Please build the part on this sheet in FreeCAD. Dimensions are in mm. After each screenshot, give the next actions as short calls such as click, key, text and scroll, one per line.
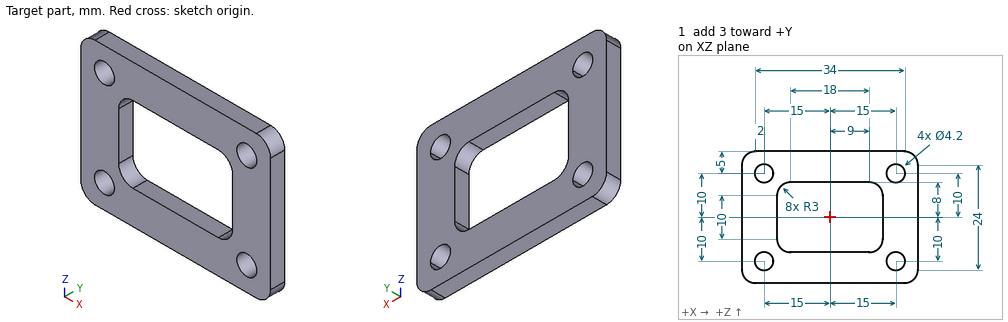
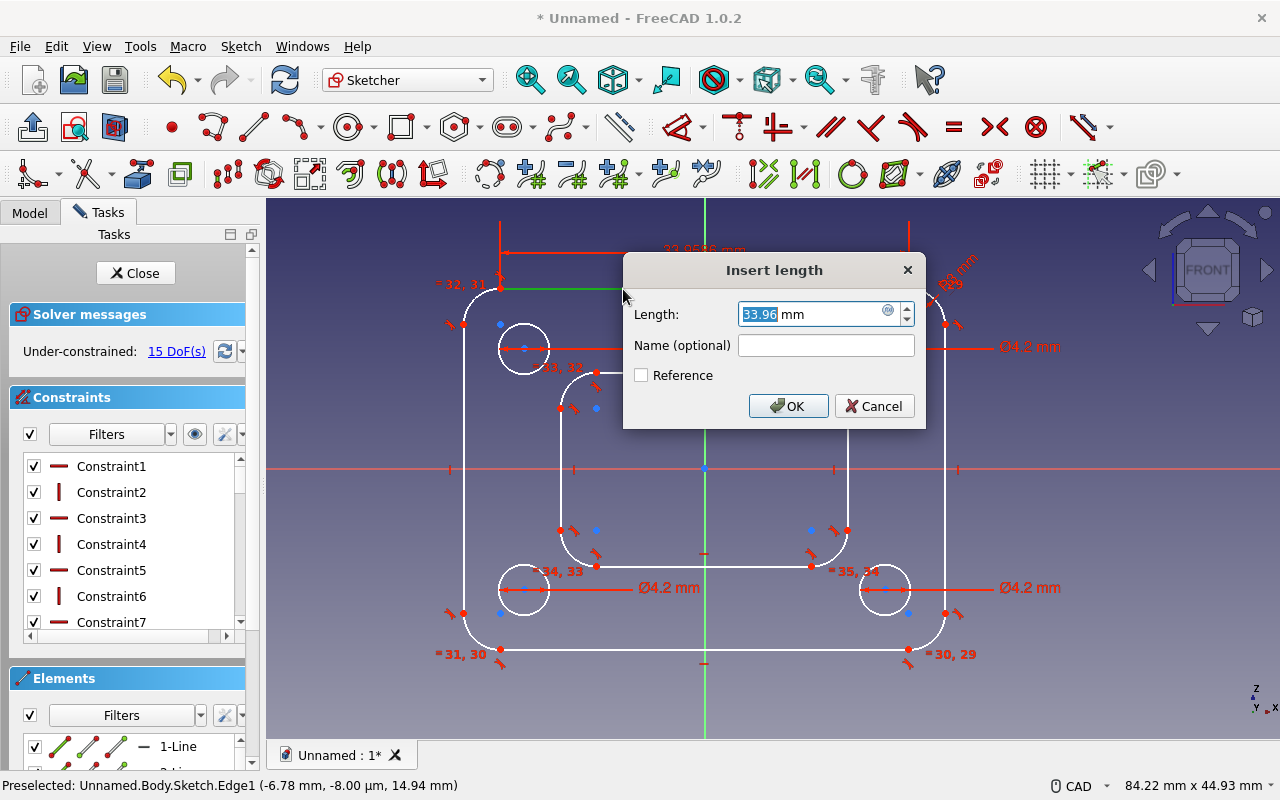
text(34)
key(Return)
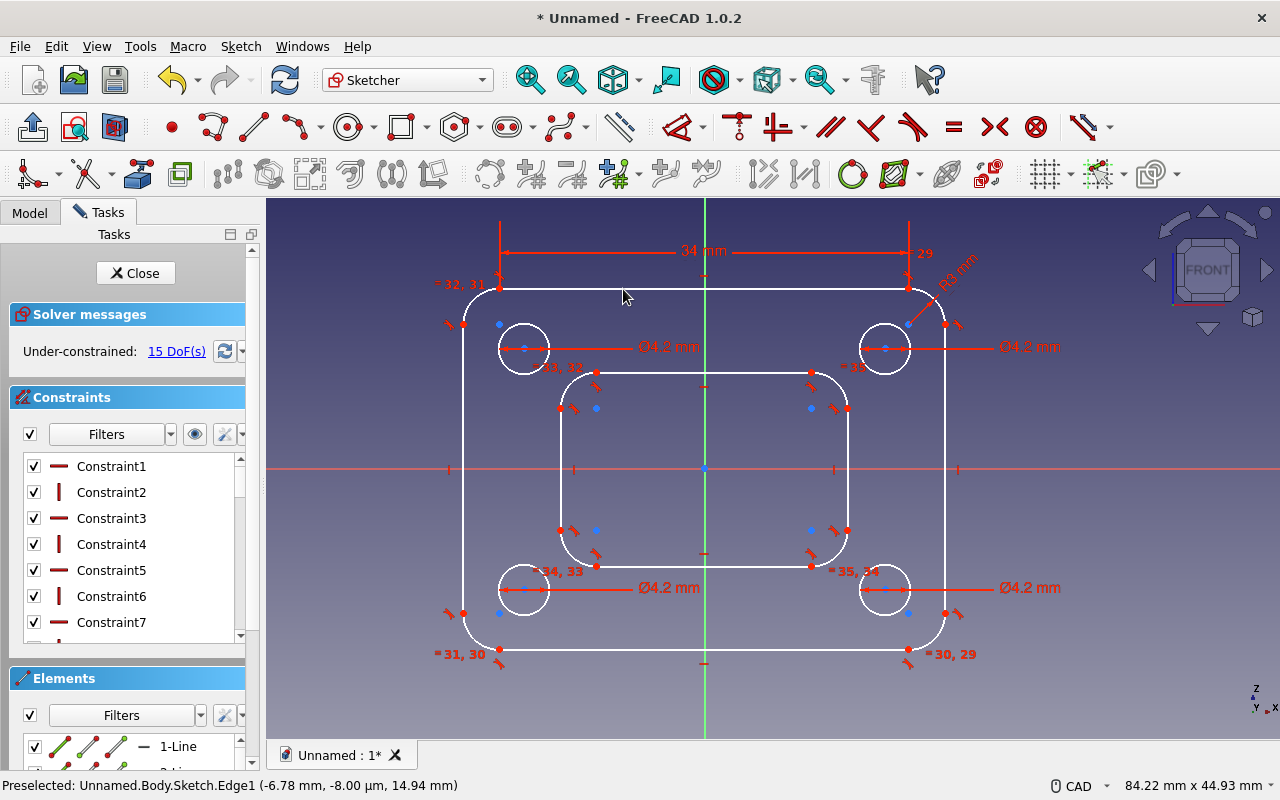
click(945, 412)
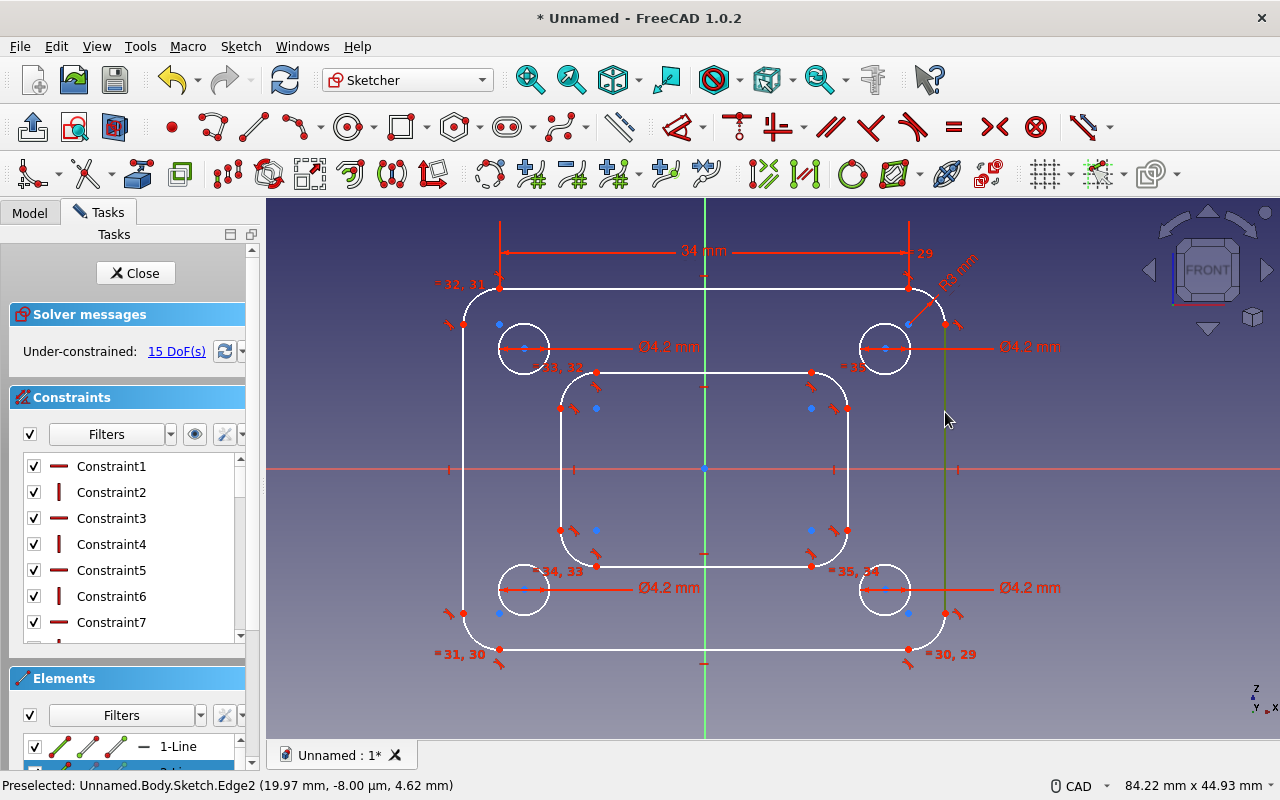
key(i)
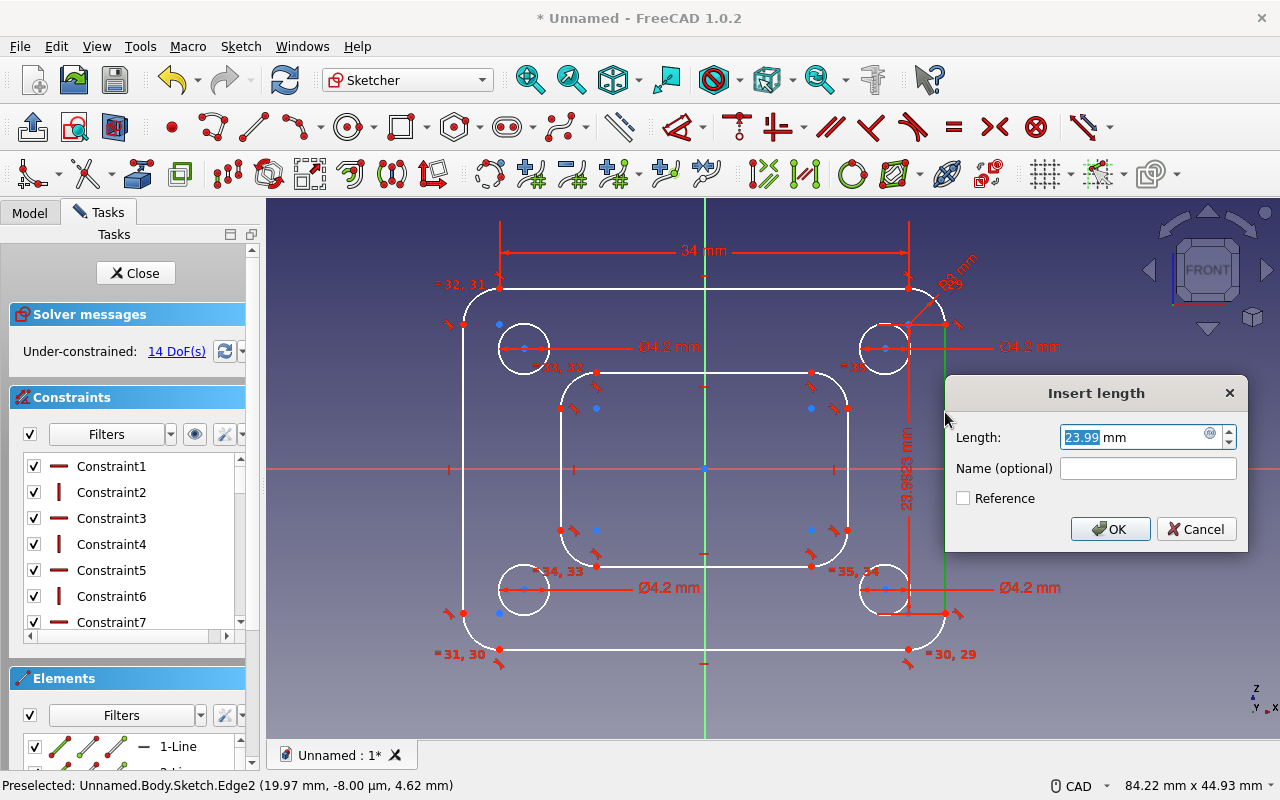
text(24)
key(Return)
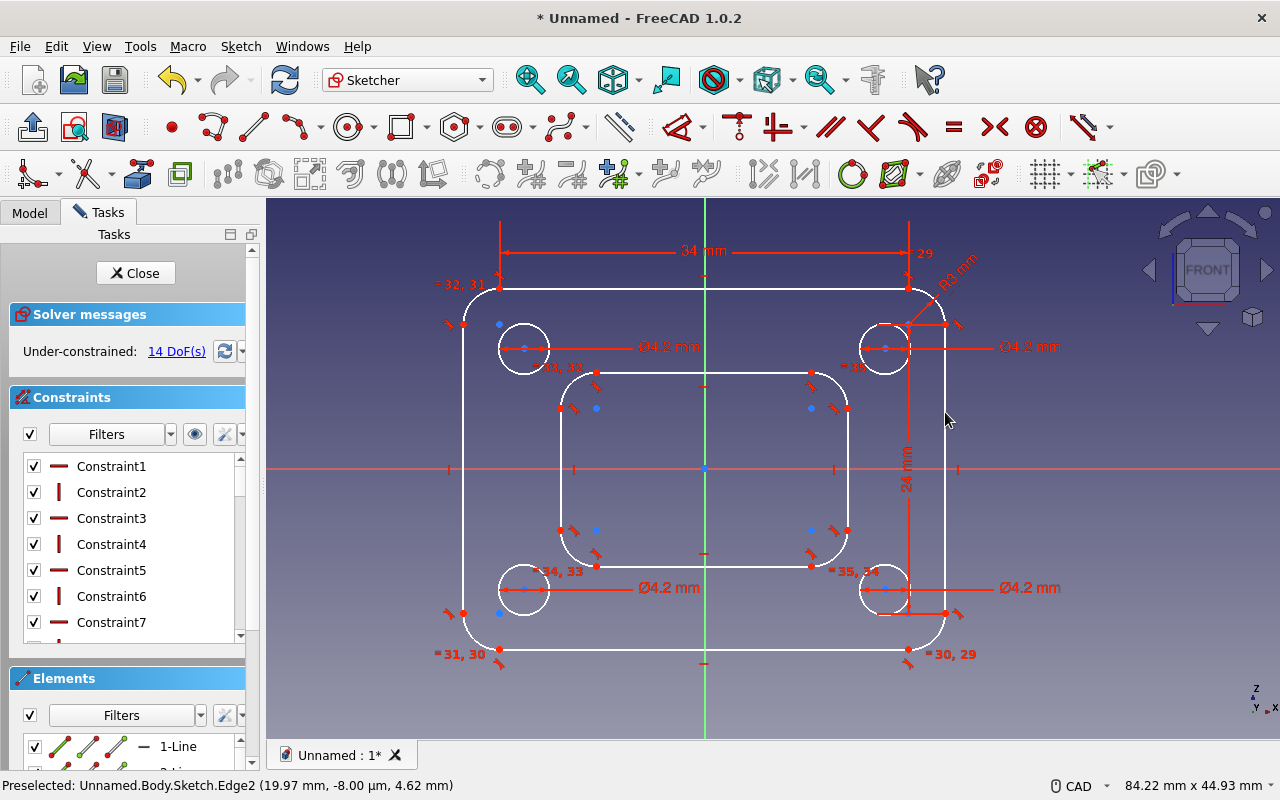
click(747, 373)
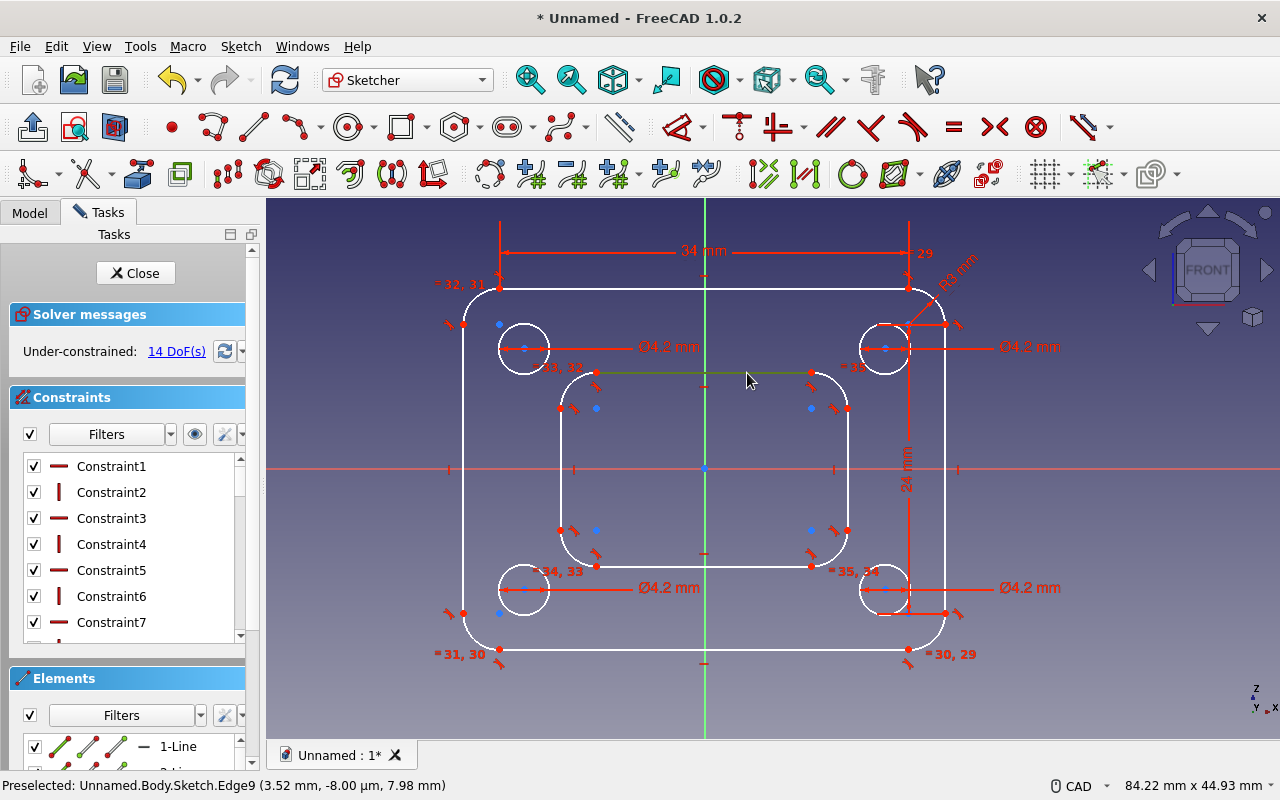
key(l)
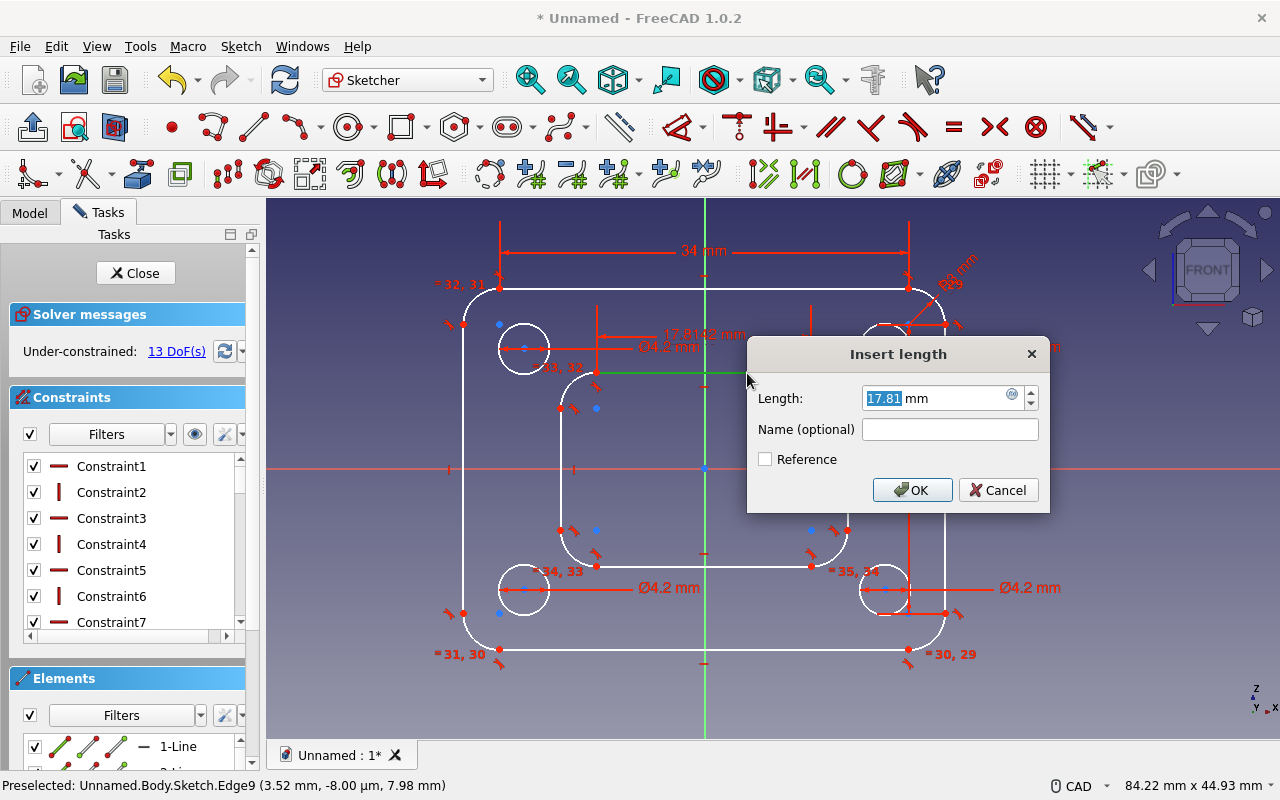
text(18)
key(Return)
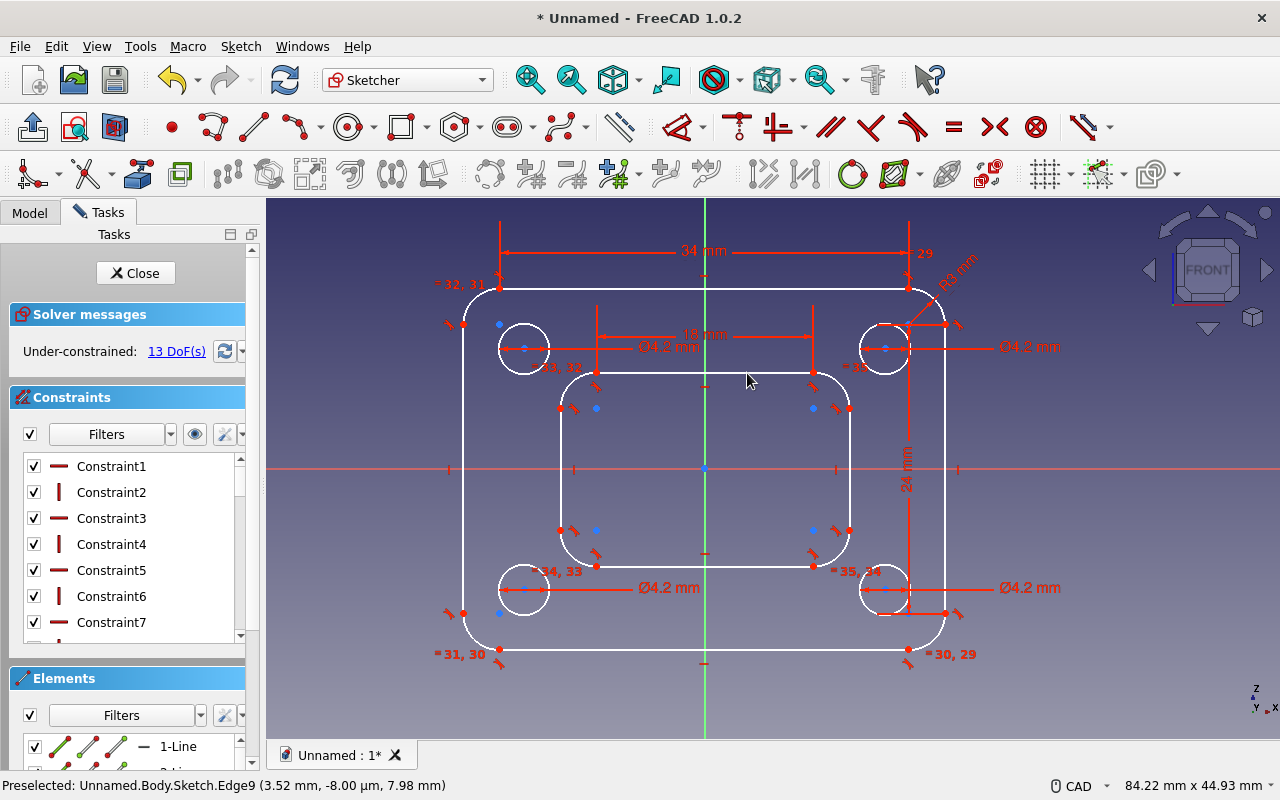
click(561, 445)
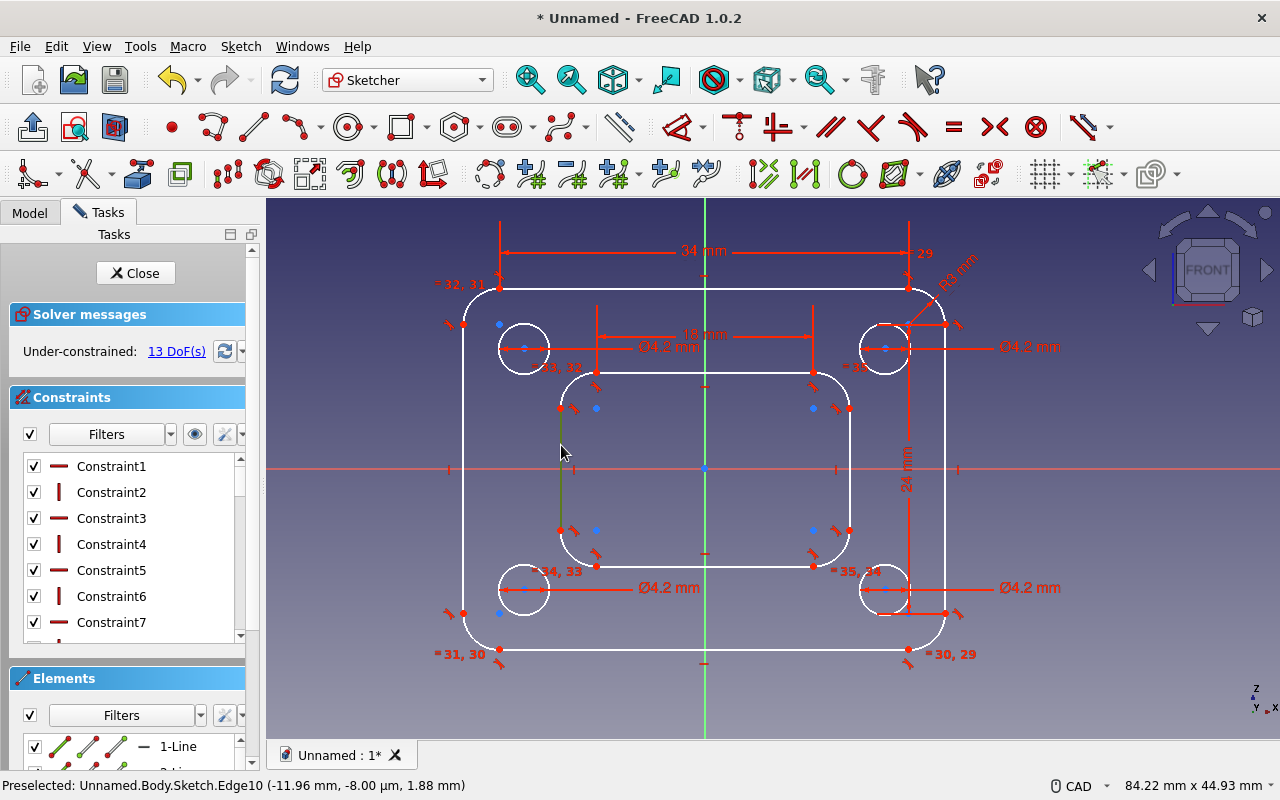
key(i)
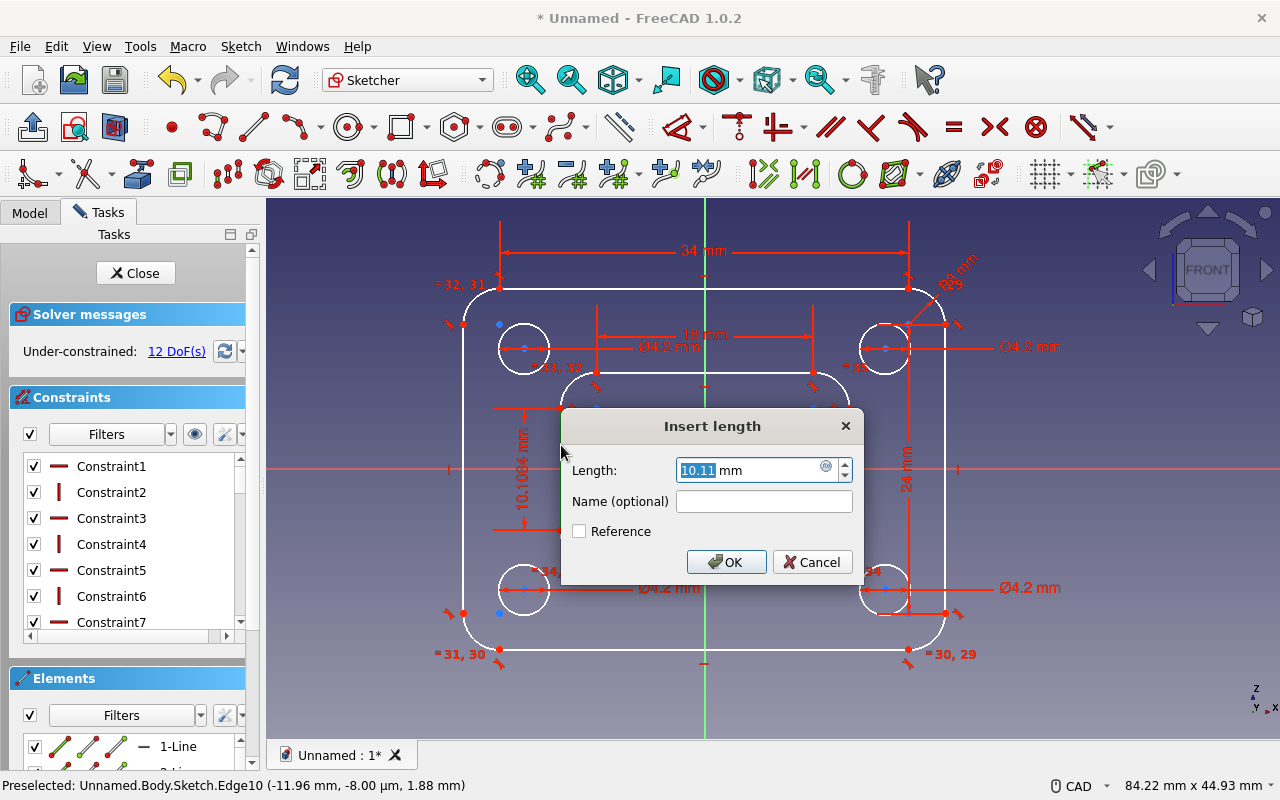
text(10)
key(Return)